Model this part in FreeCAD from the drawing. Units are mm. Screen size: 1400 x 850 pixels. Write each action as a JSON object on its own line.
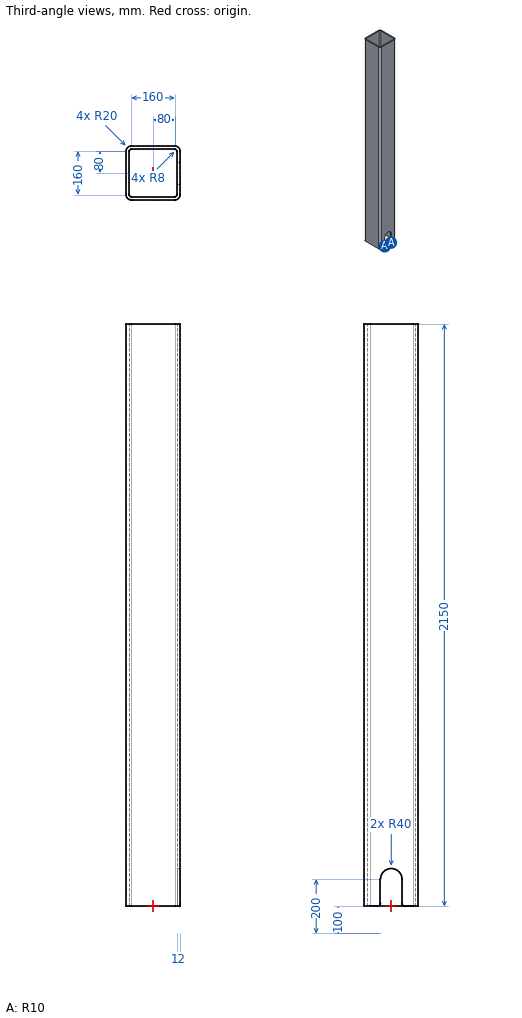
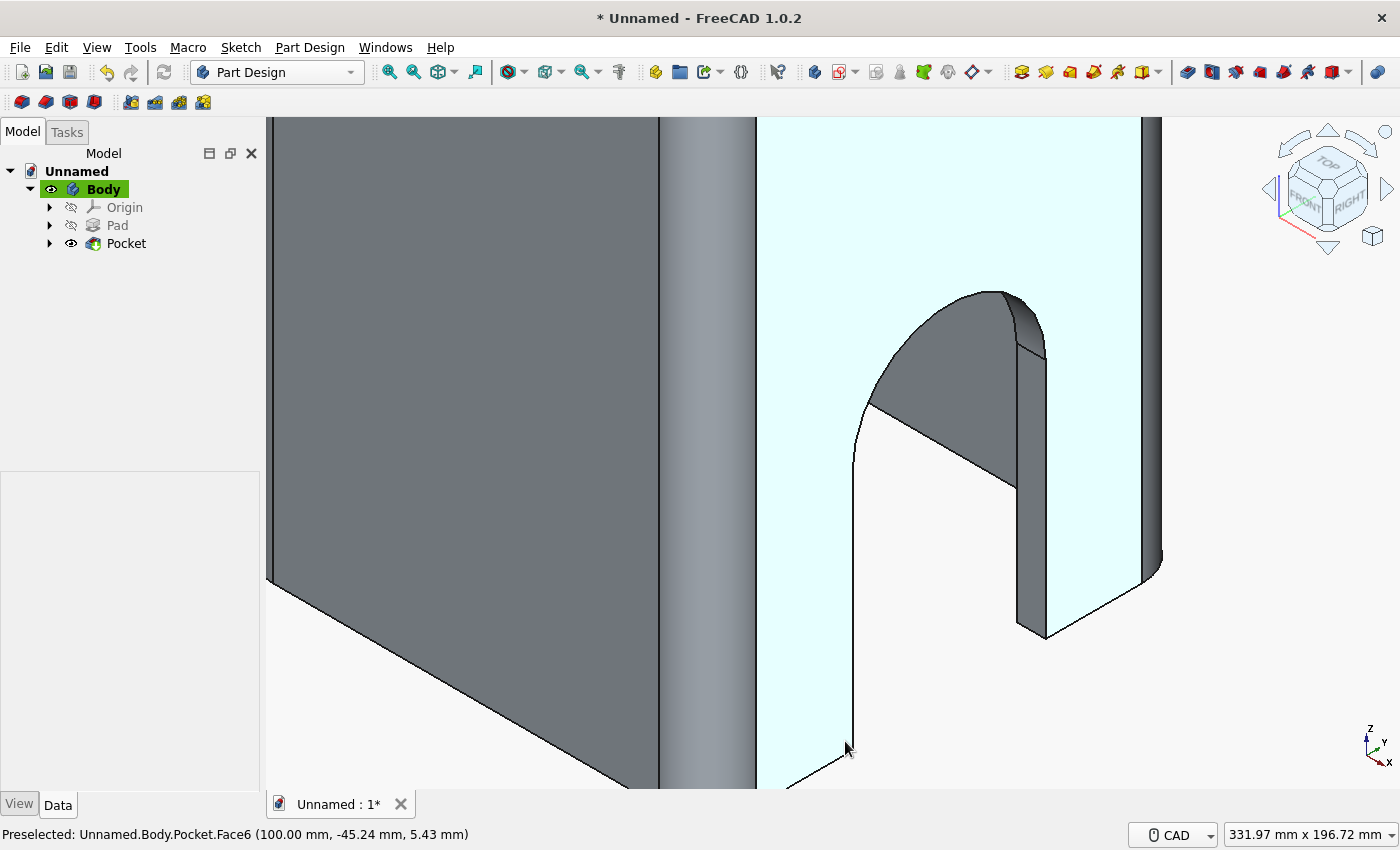
{"action": "left_click", "coordinate": [390, 72]}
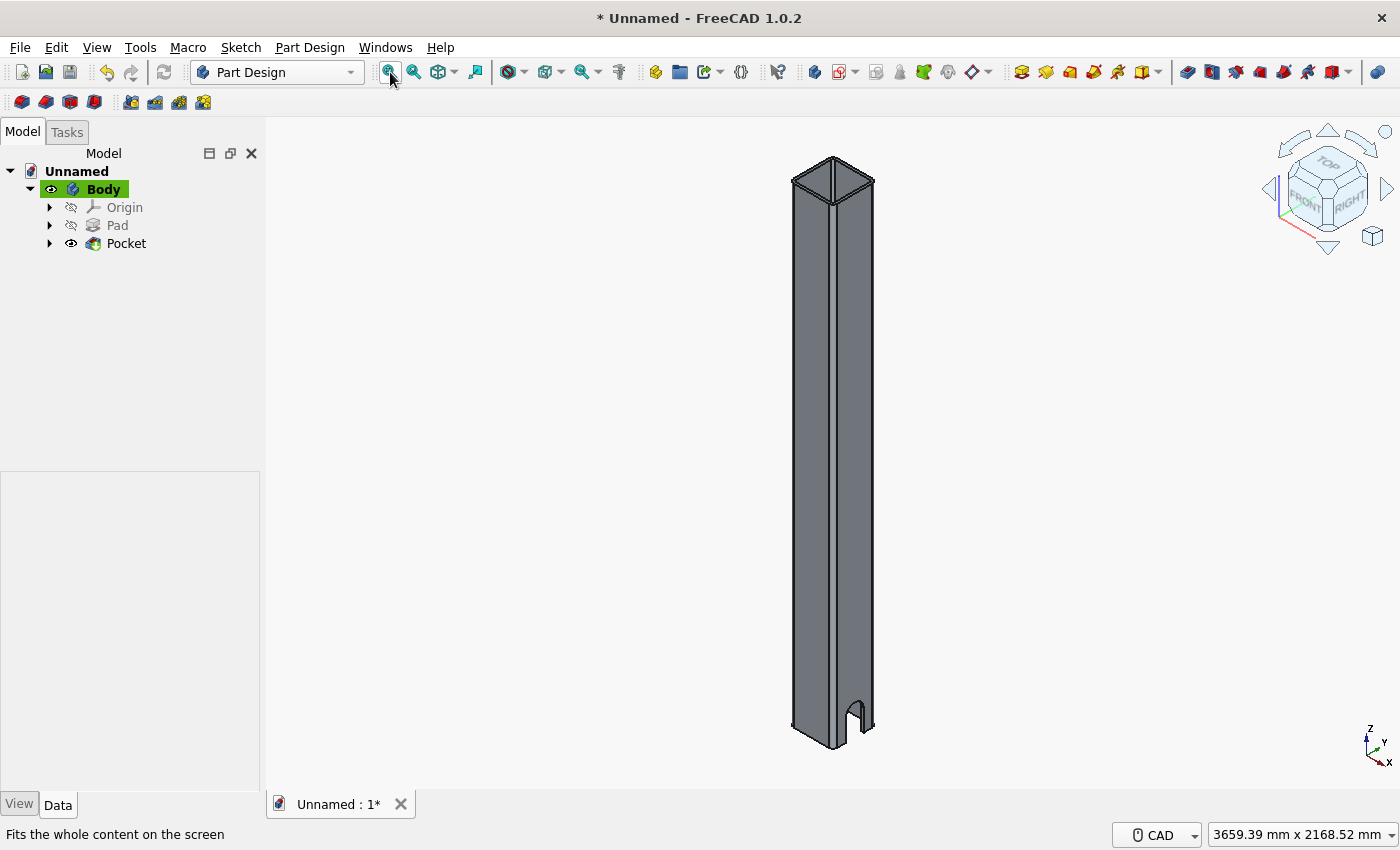
{"action": "key", "text": "2"}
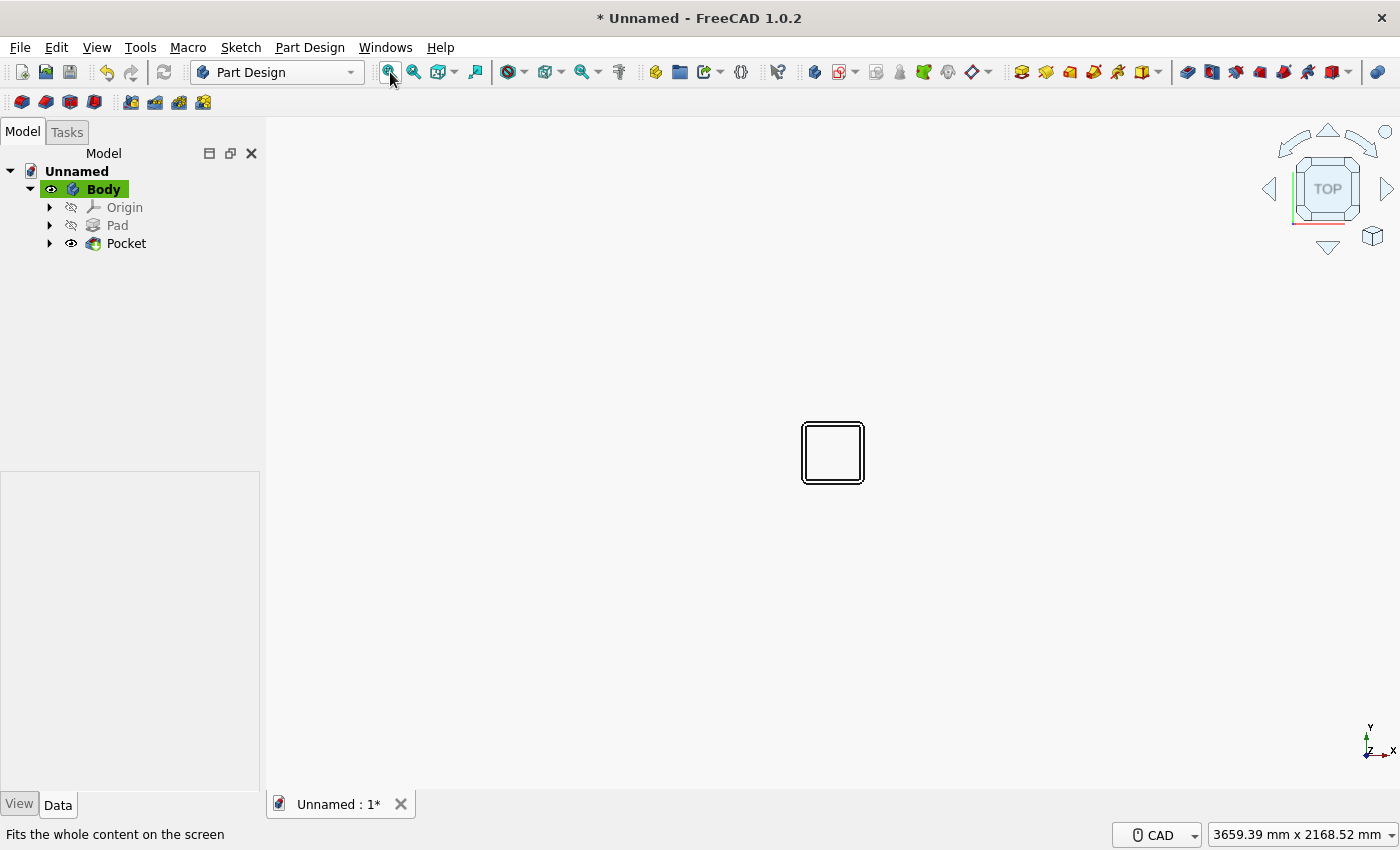
{"action": "left_click", "coordinate": [390, 72]}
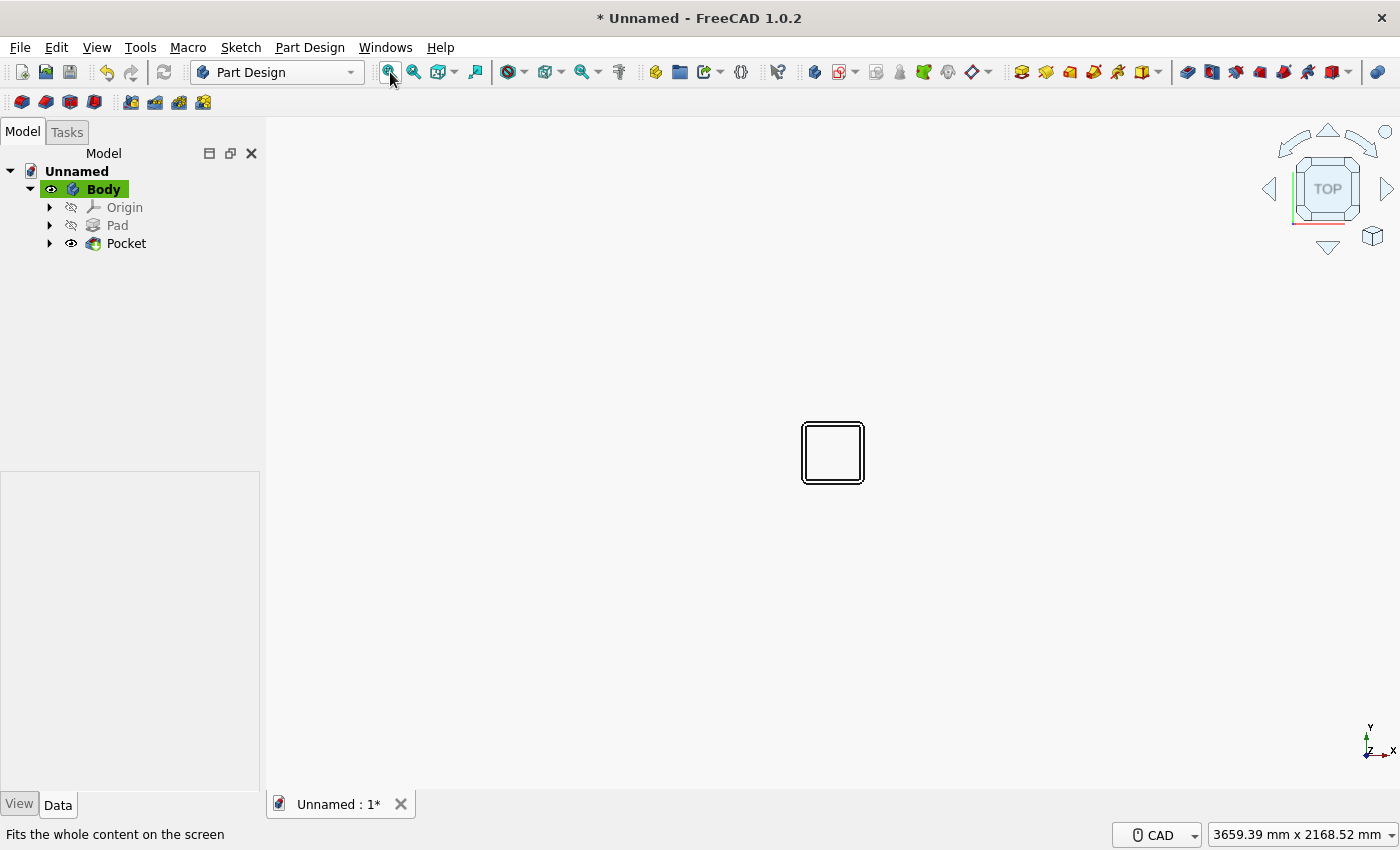
{"action": "scroll", "coordinate": [862, 464], "scroll_direction": "up", "scroll_amount": 12}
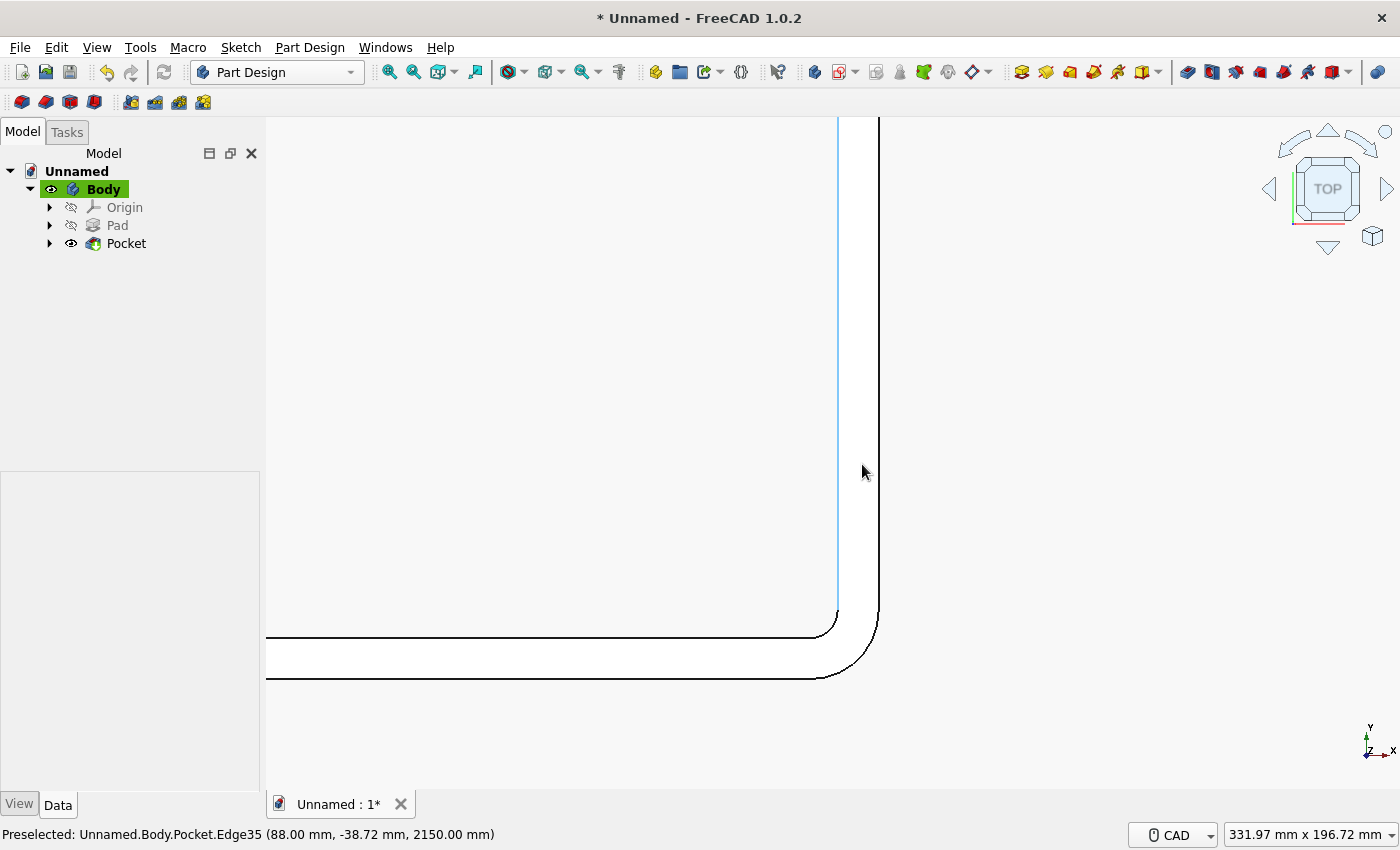
{"action": "left_click", "coordinate": [390, 72]}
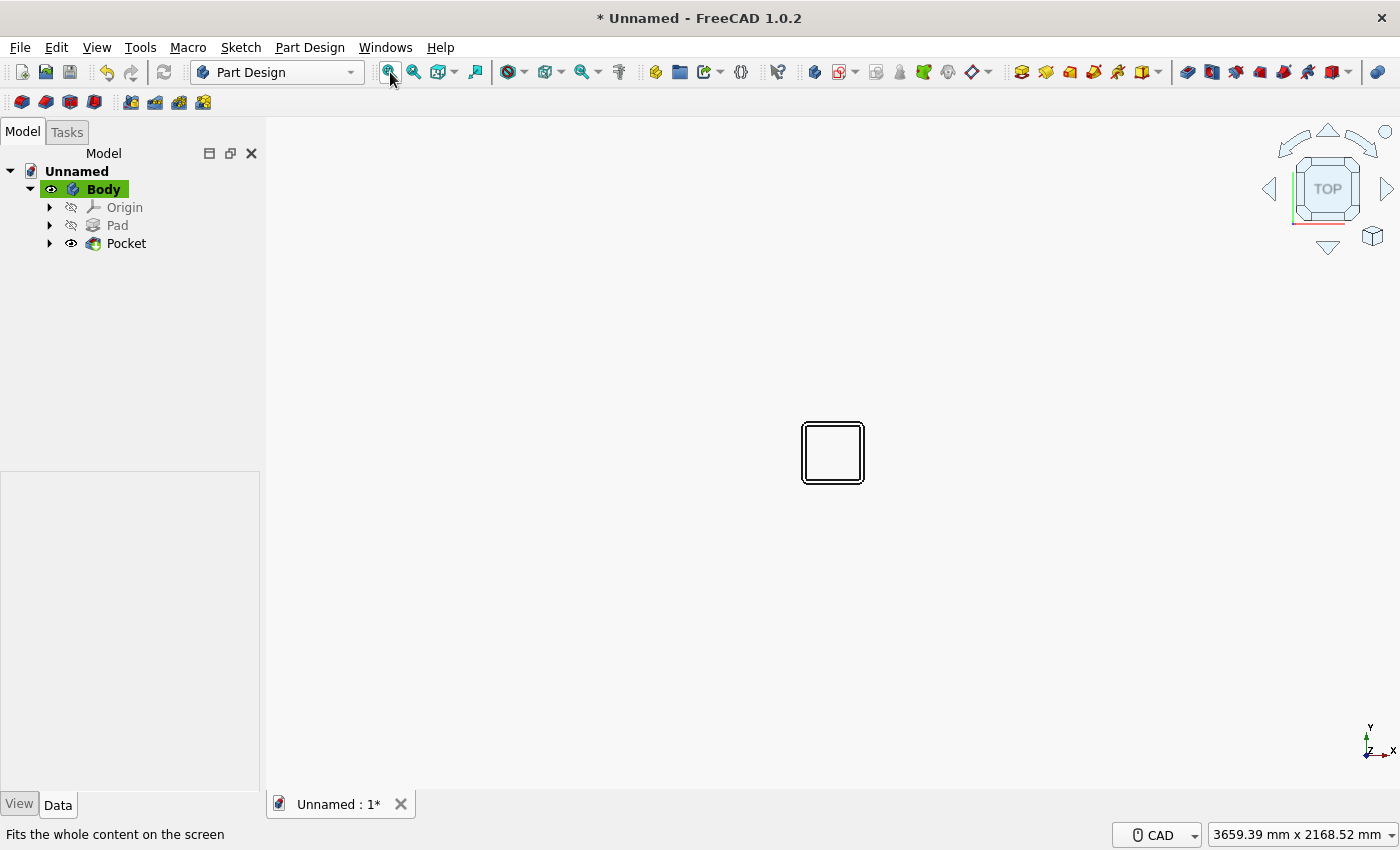
{"action": "key", "text": "1"}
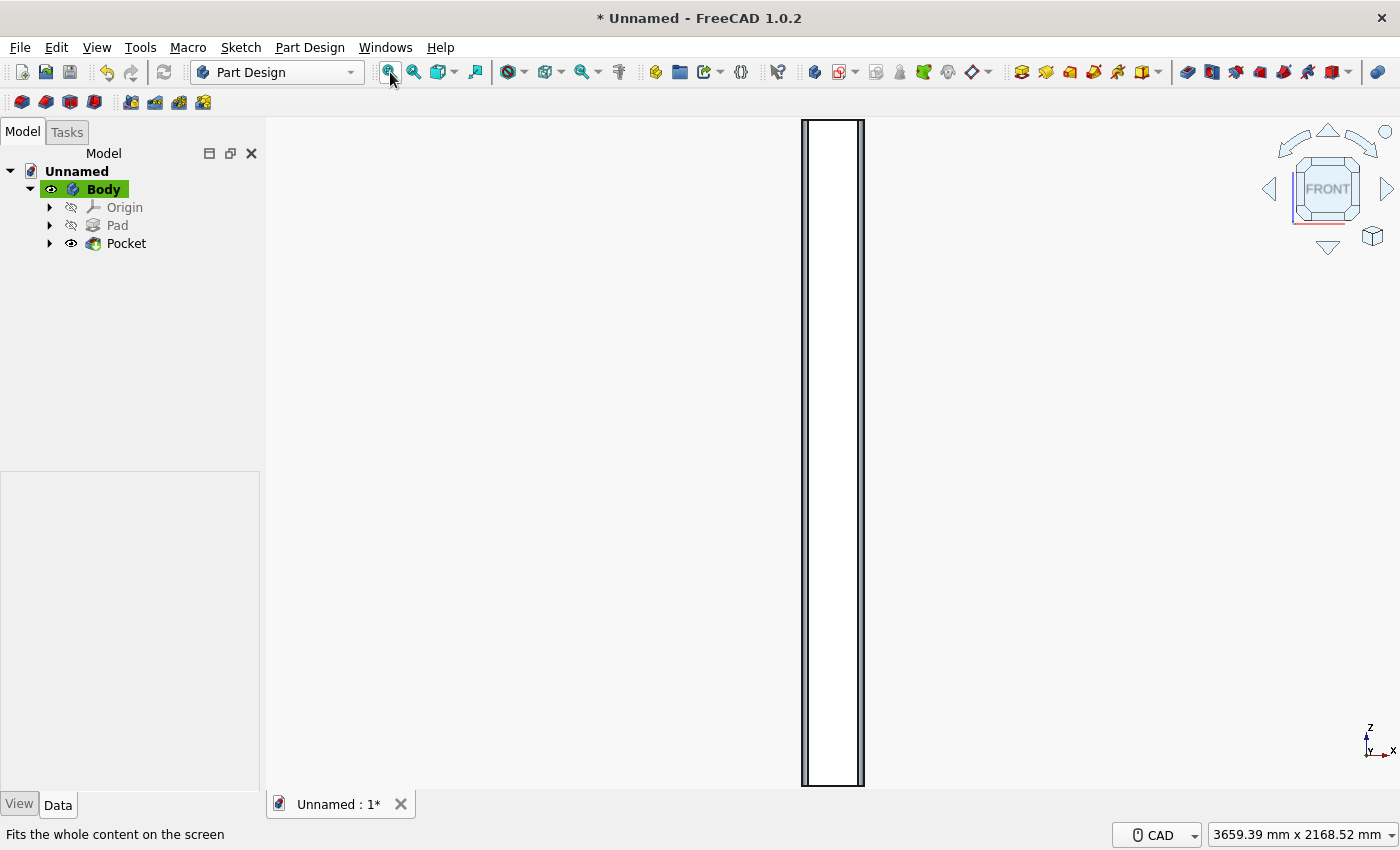
{"action": "key", "text": "3"}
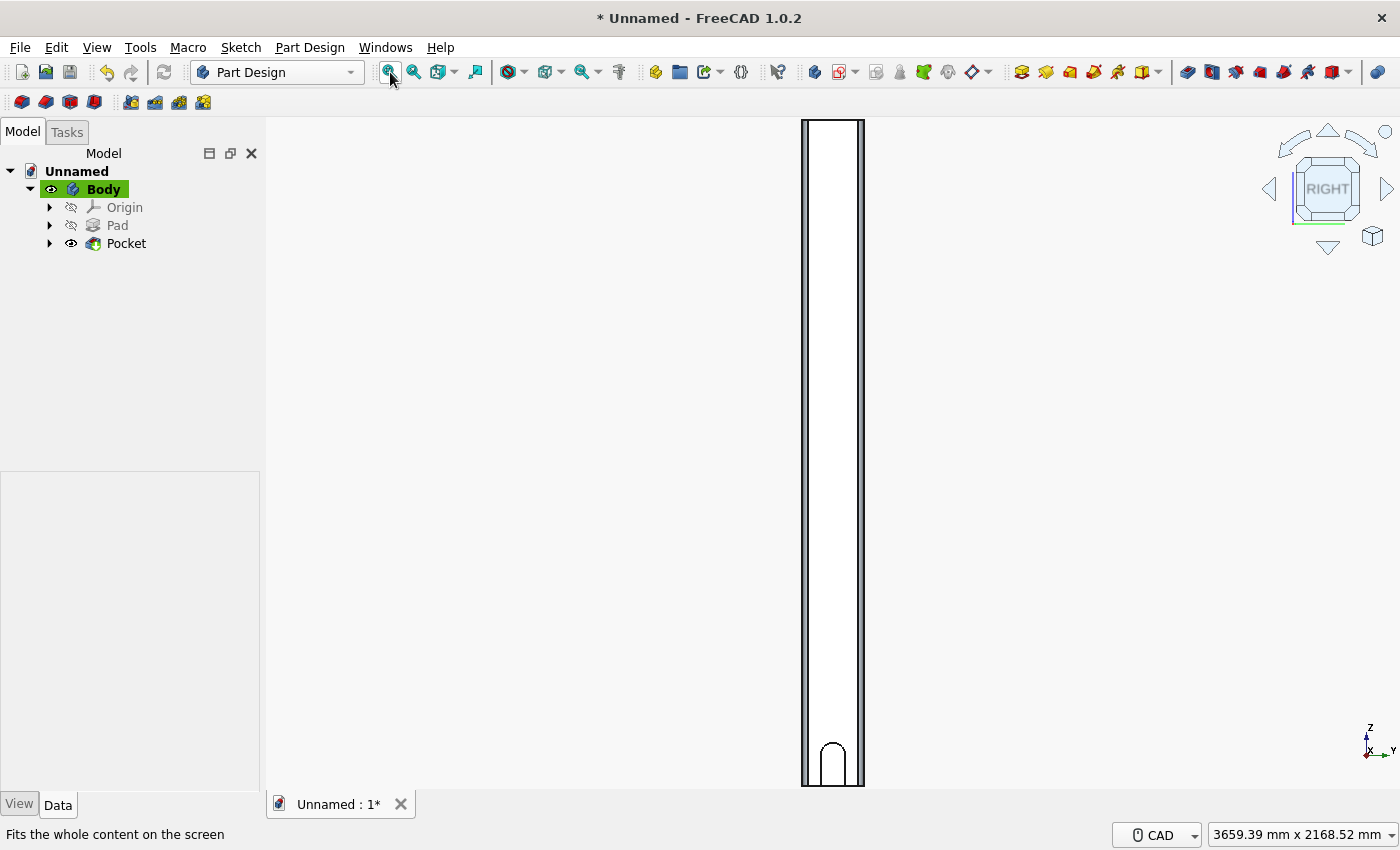
{"action": "key", "text": "5"}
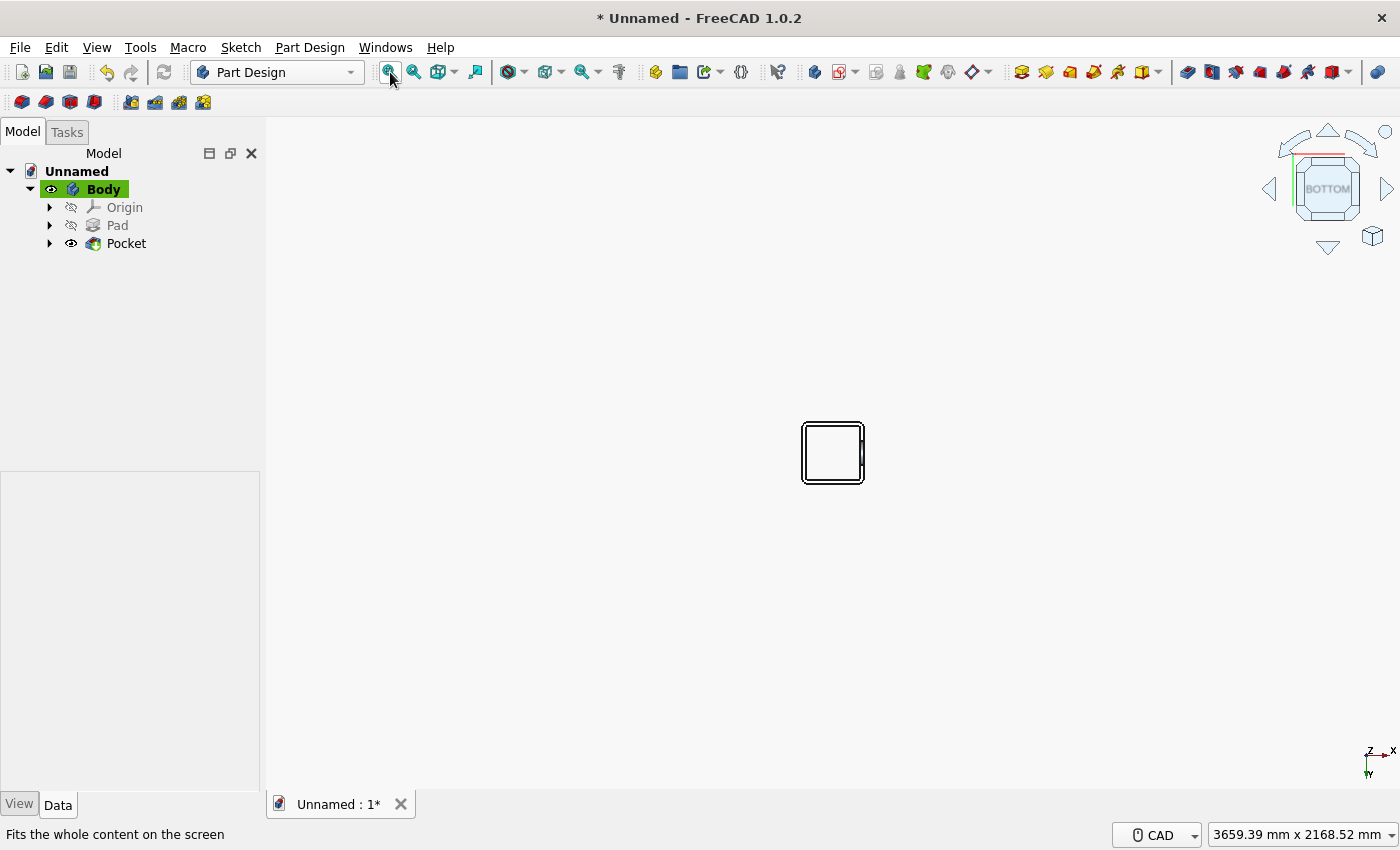
{"action": "left_click", "coordinate": [390, 72]}